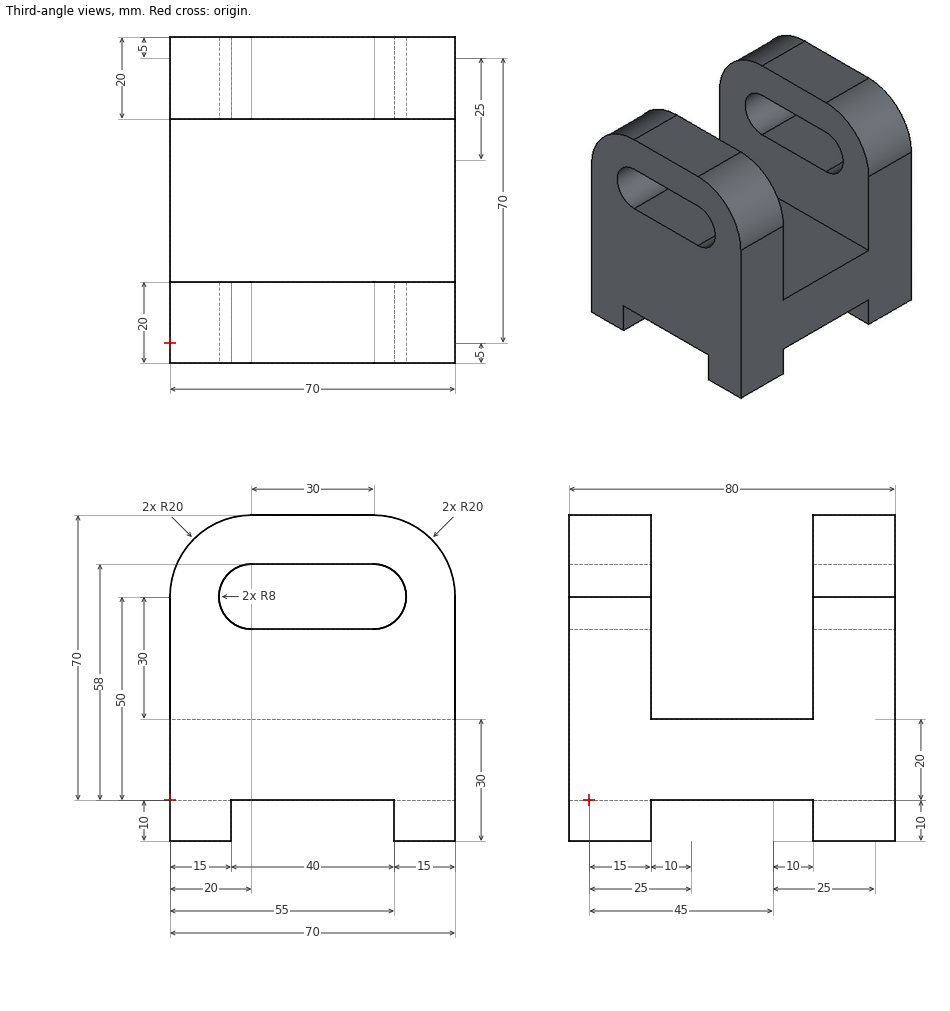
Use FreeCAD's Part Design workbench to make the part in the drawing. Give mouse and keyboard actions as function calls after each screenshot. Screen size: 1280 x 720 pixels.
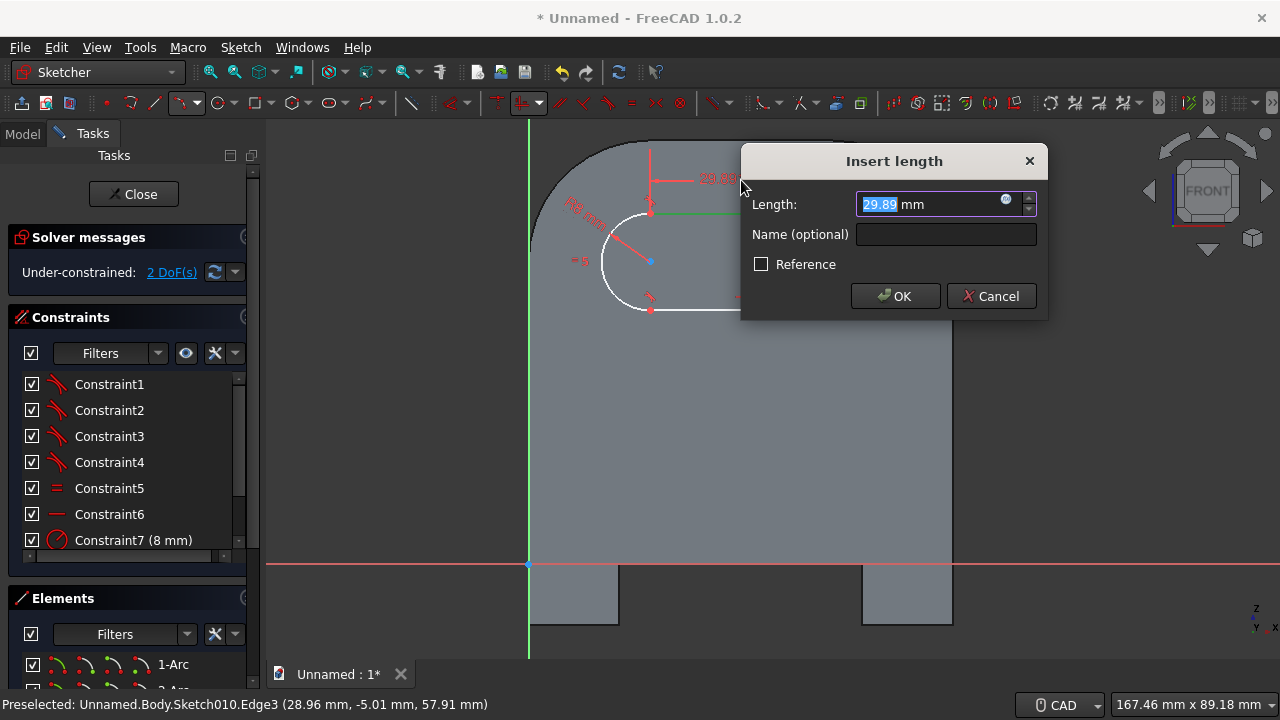
text(30)
key(Return)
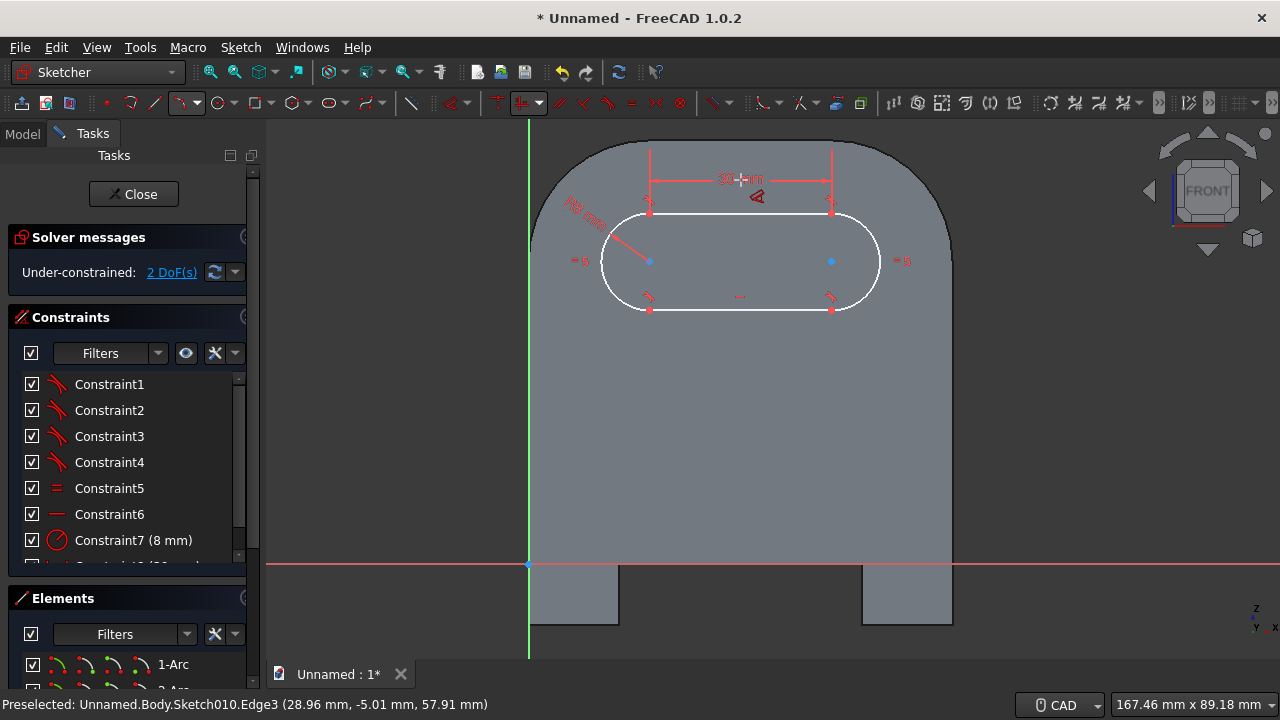
click(650, 214)
click(589, 598)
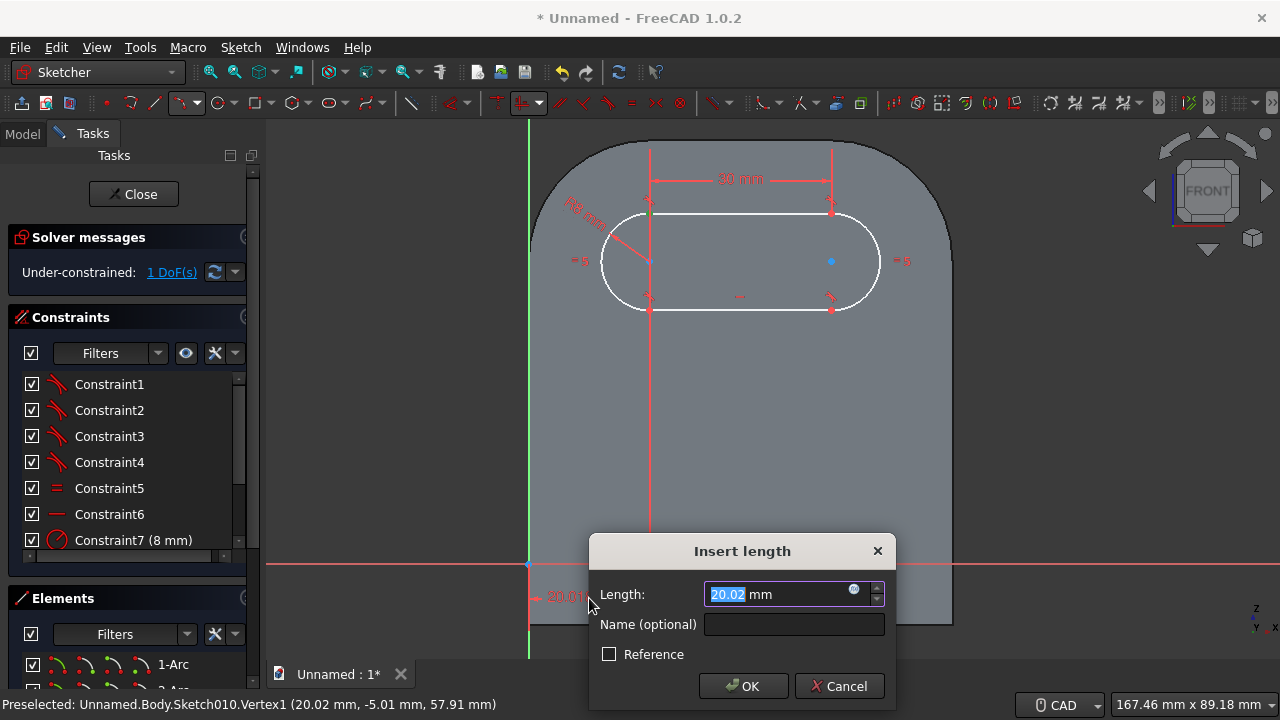
text(20)
key(Return)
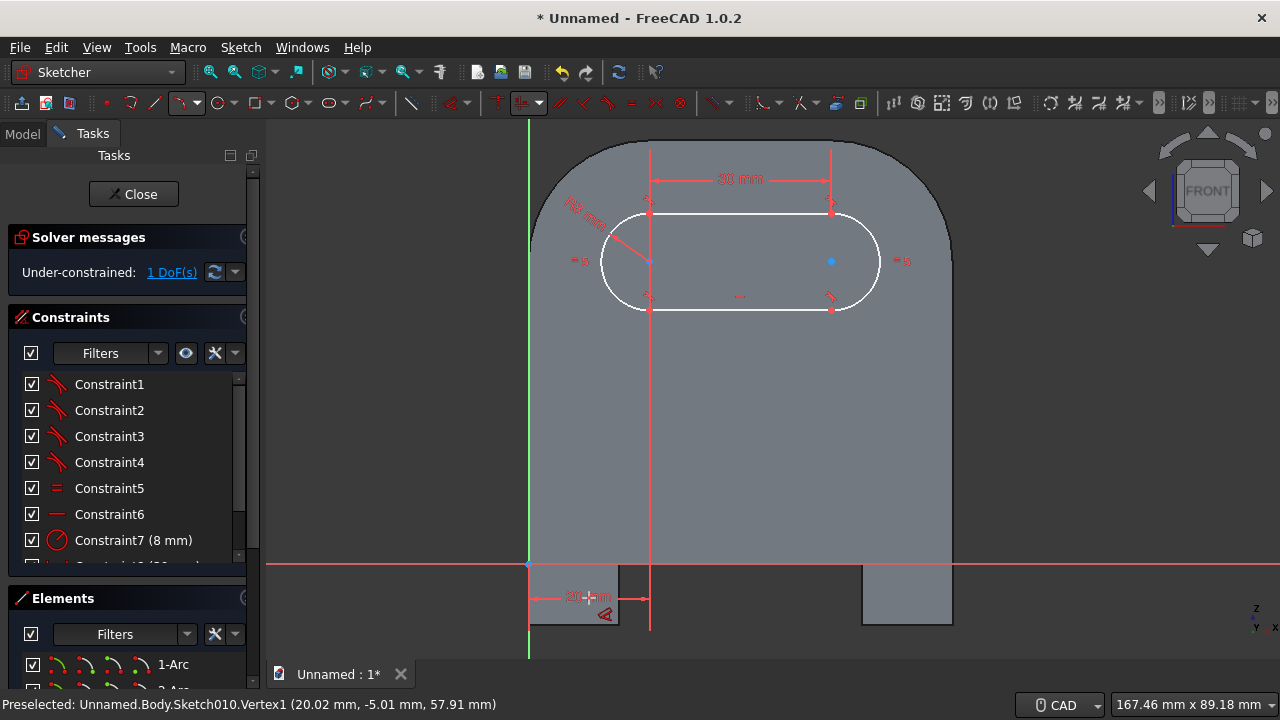
click(650, 214)
click(495, 389)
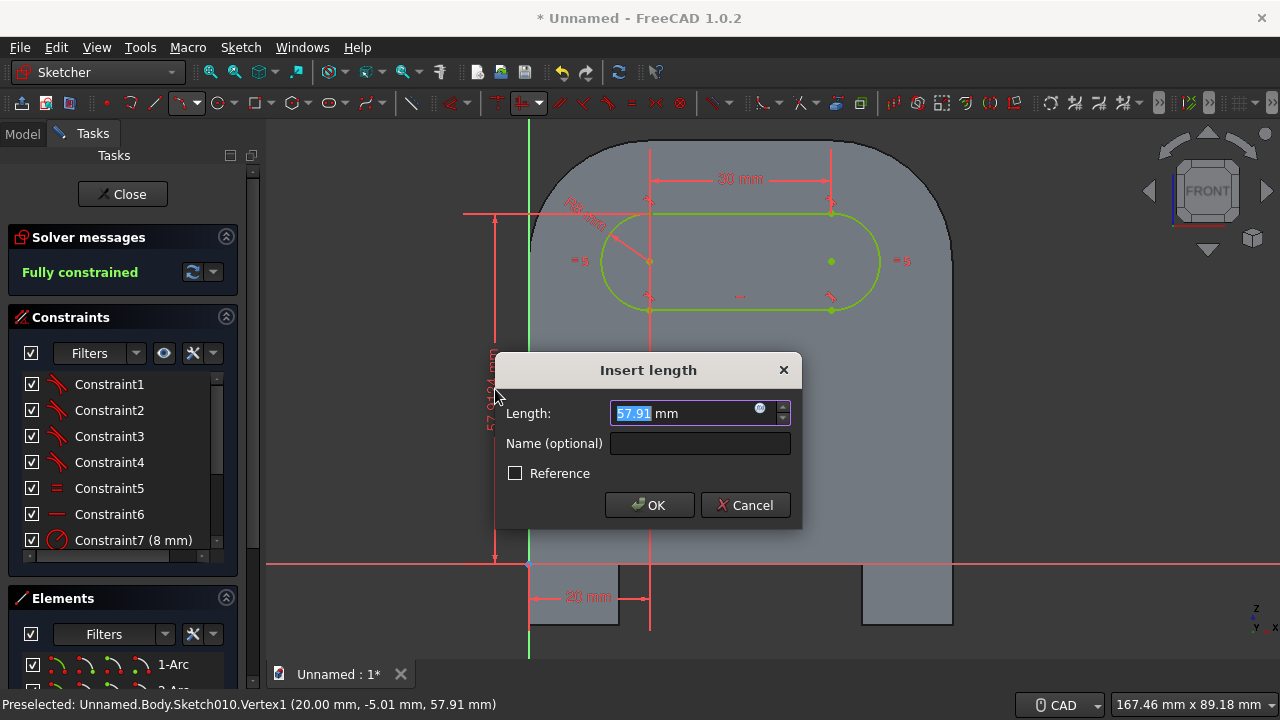
text(58)
key(Return)
key(Escape)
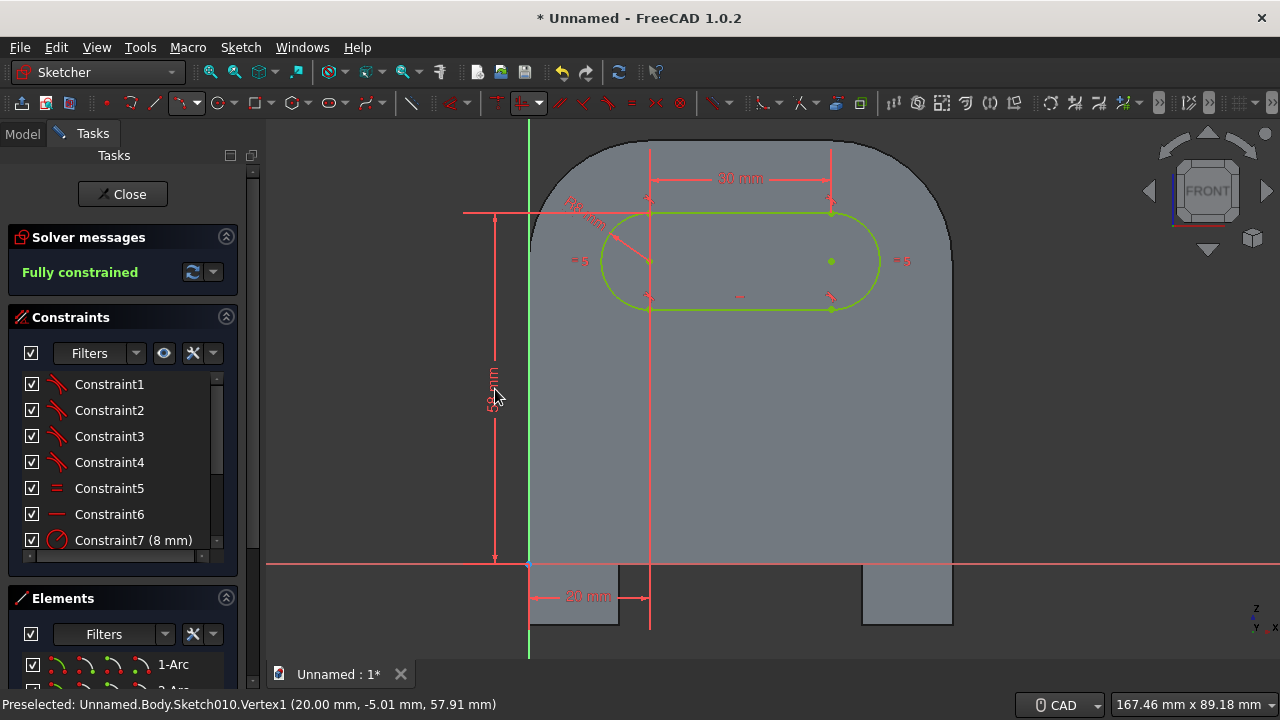
click(123, 194)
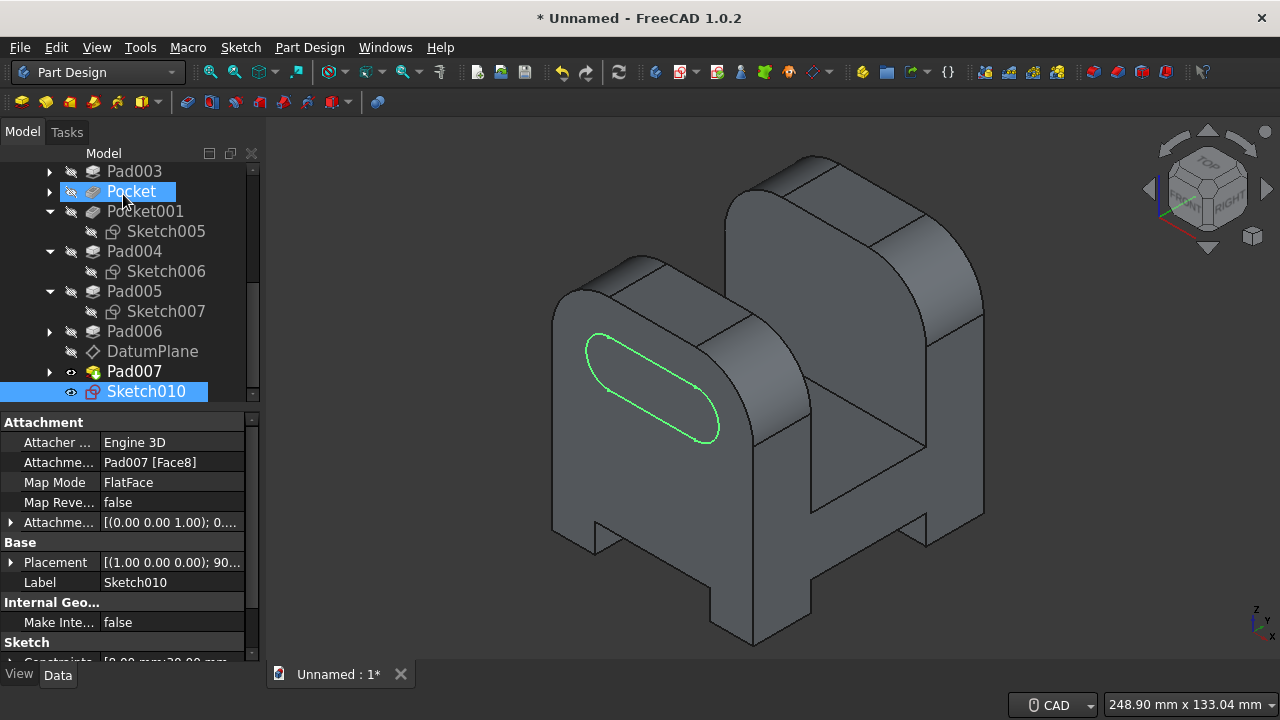
click(188, 102)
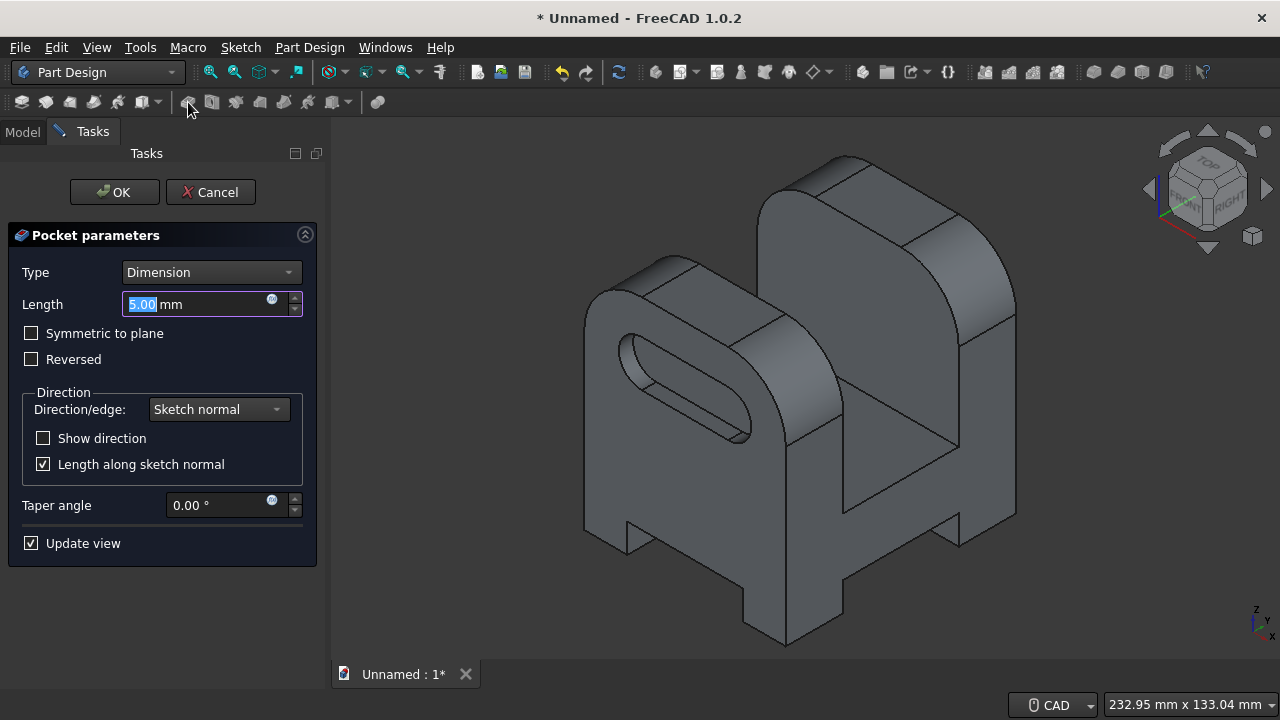
text(80)
key(Tab)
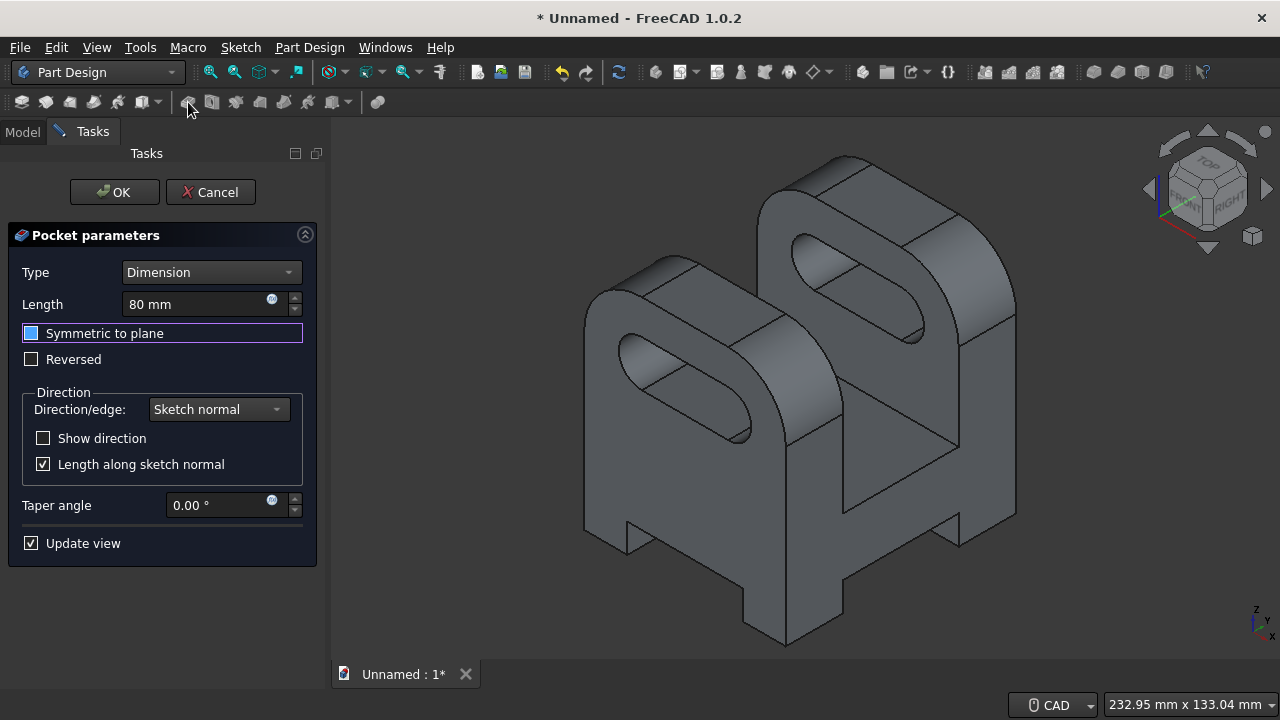
click(115, 192)